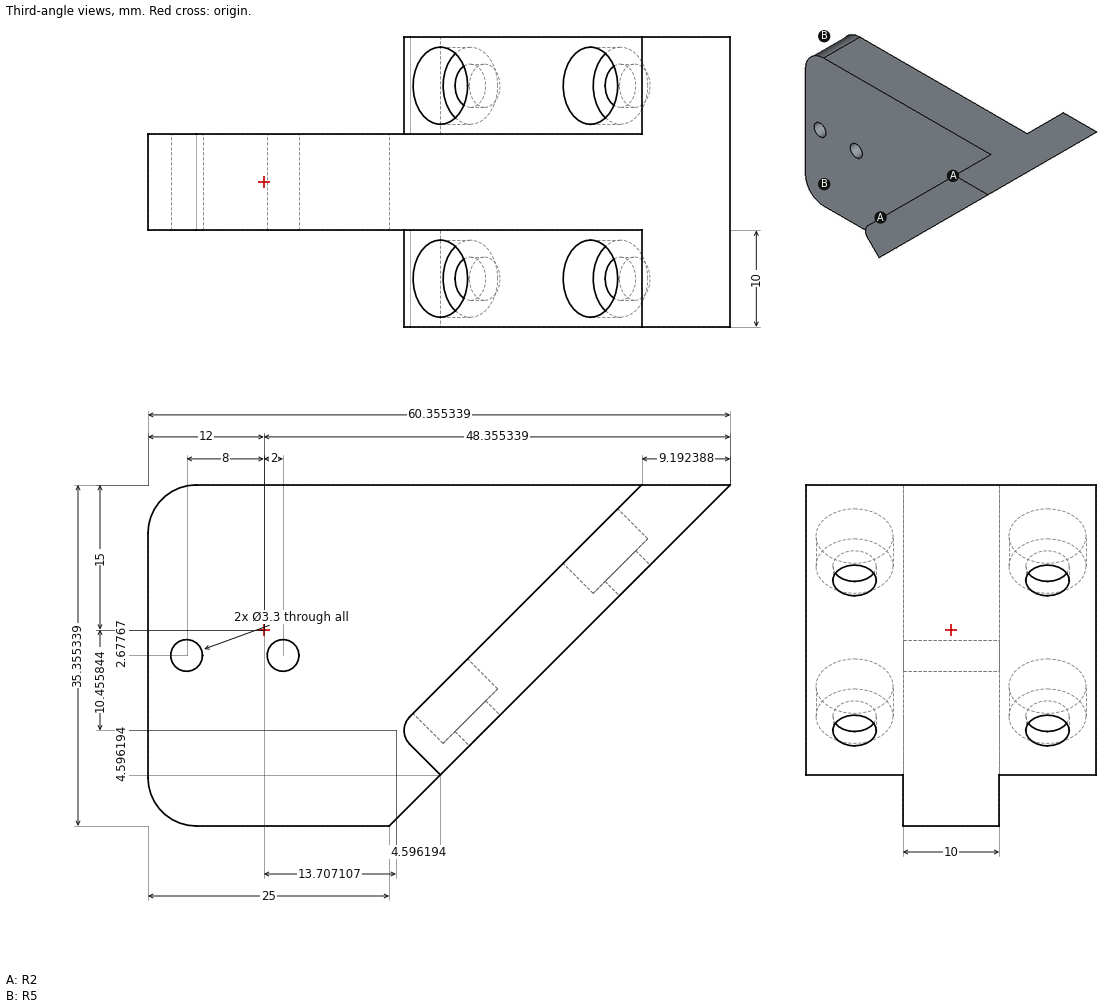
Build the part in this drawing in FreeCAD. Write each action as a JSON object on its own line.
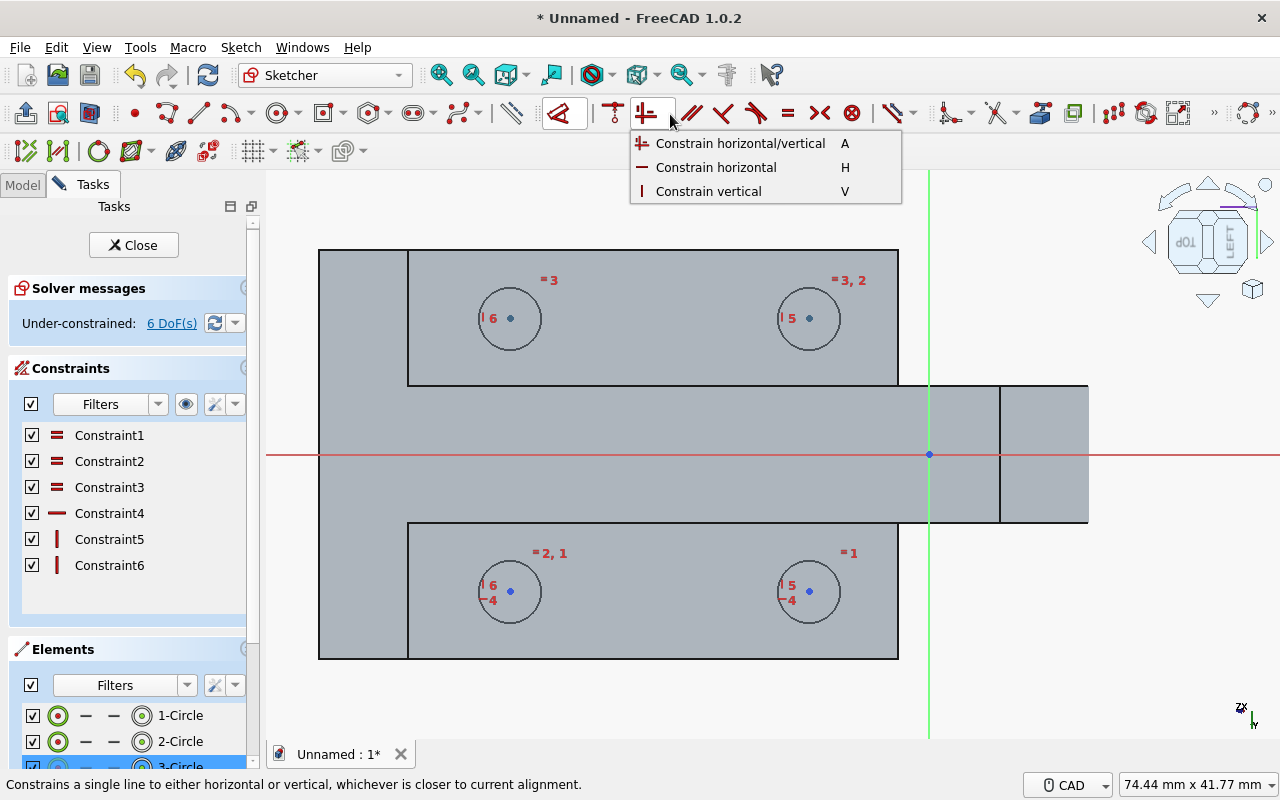
{"action": "left_click", "coordinate": [766, 167]}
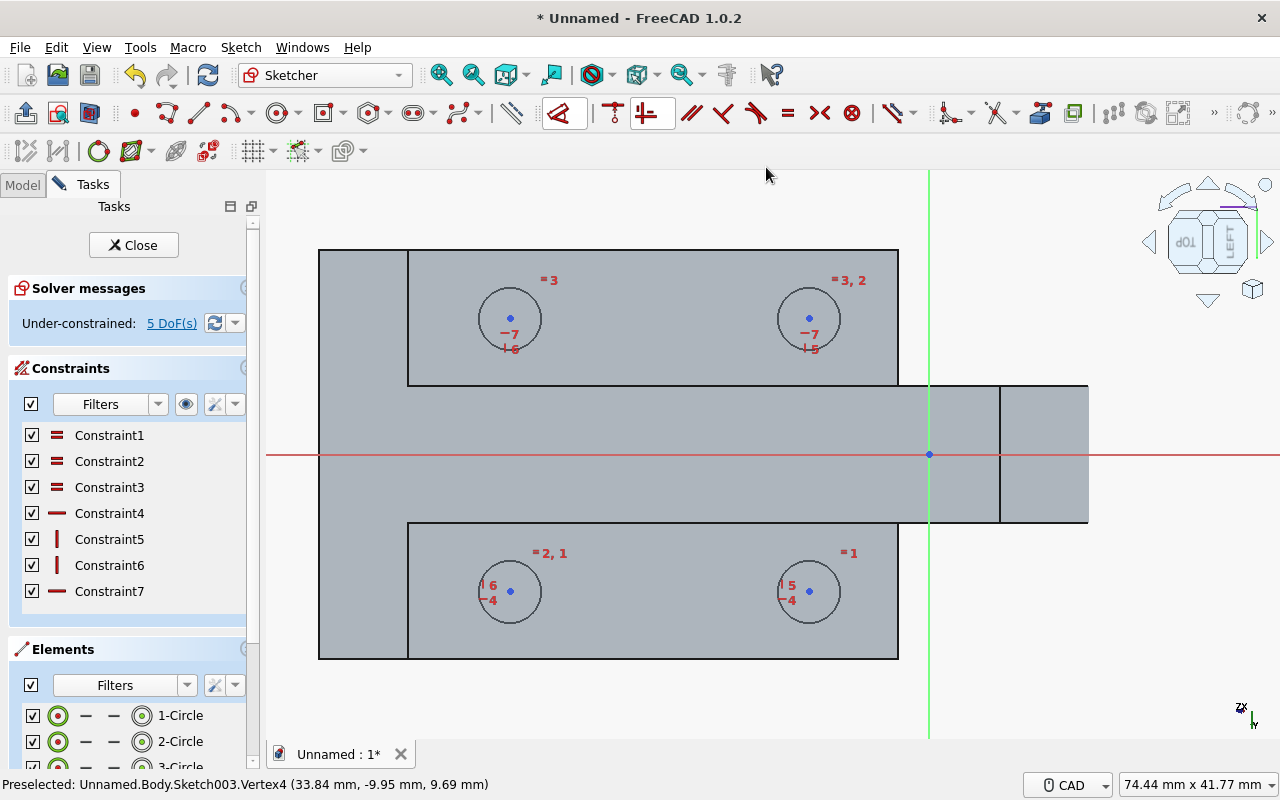
{"action": "left_click", "coordinate": [831, 570]}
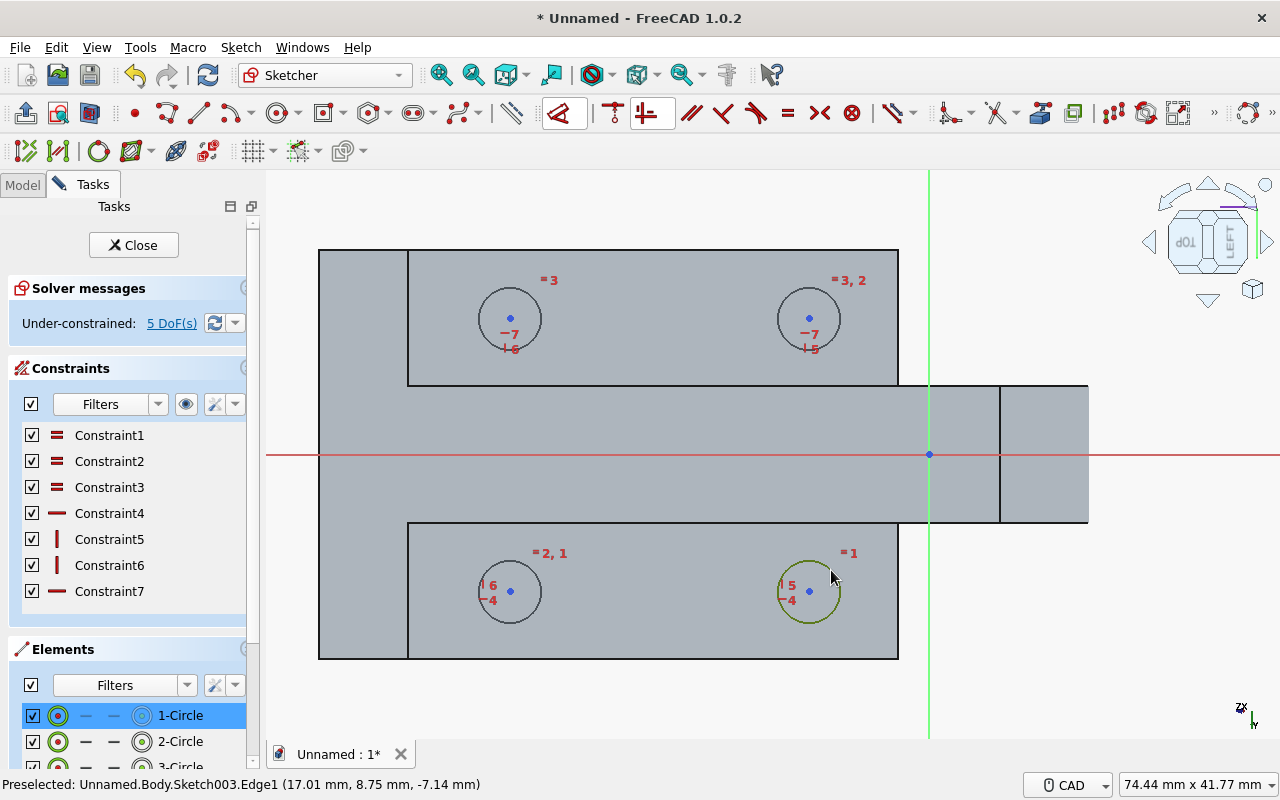
{"action": "key", "text": "k o"}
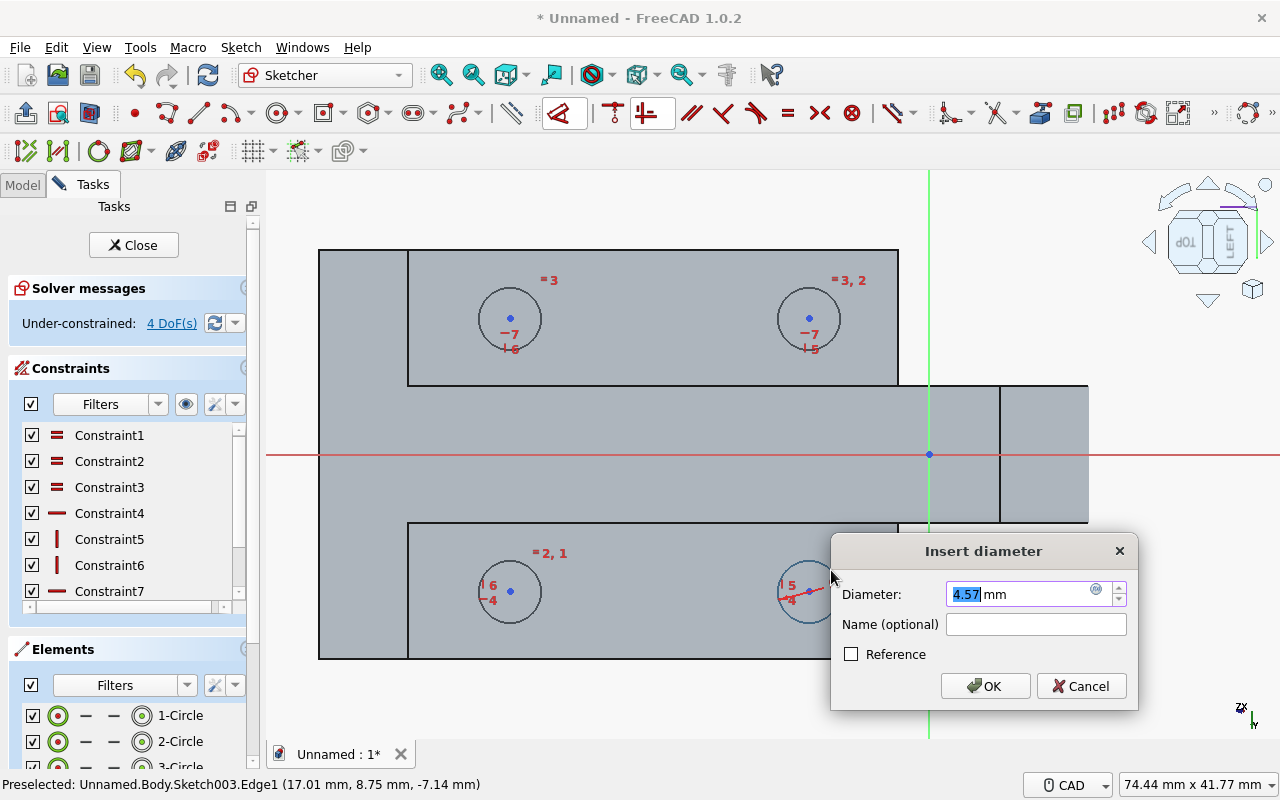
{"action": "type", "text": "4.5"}
{"action": "key", "text": "Return"}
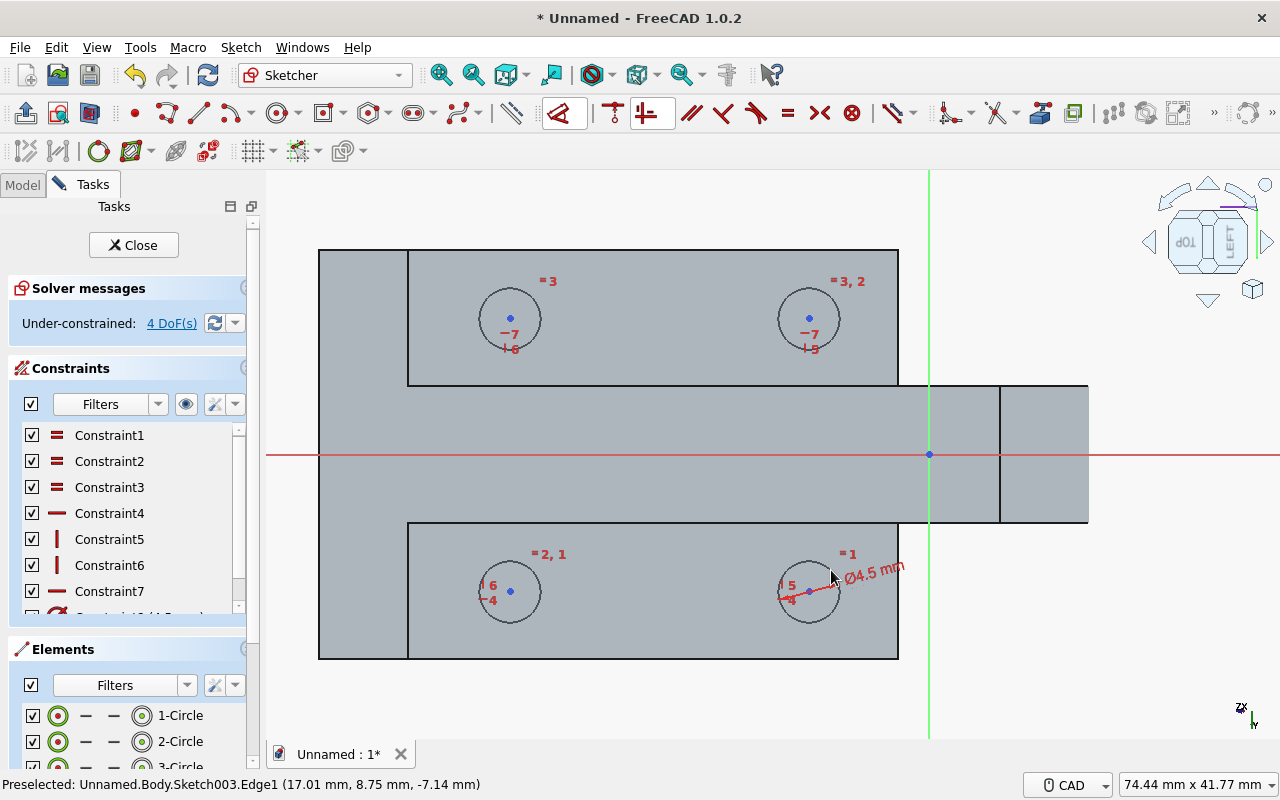
{"action": "left_click", "coordinate": [809, 592]}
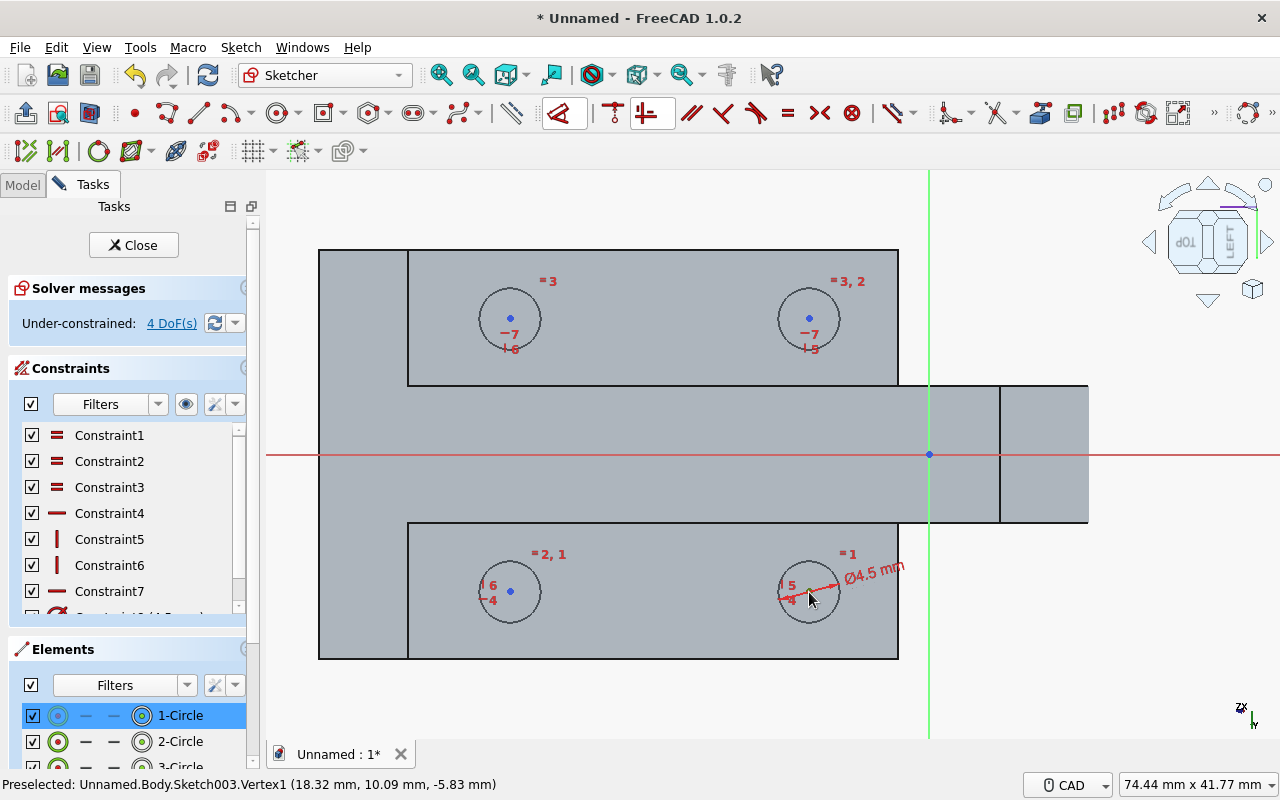
{"action": "left_click", "coordinate": [582, 114]}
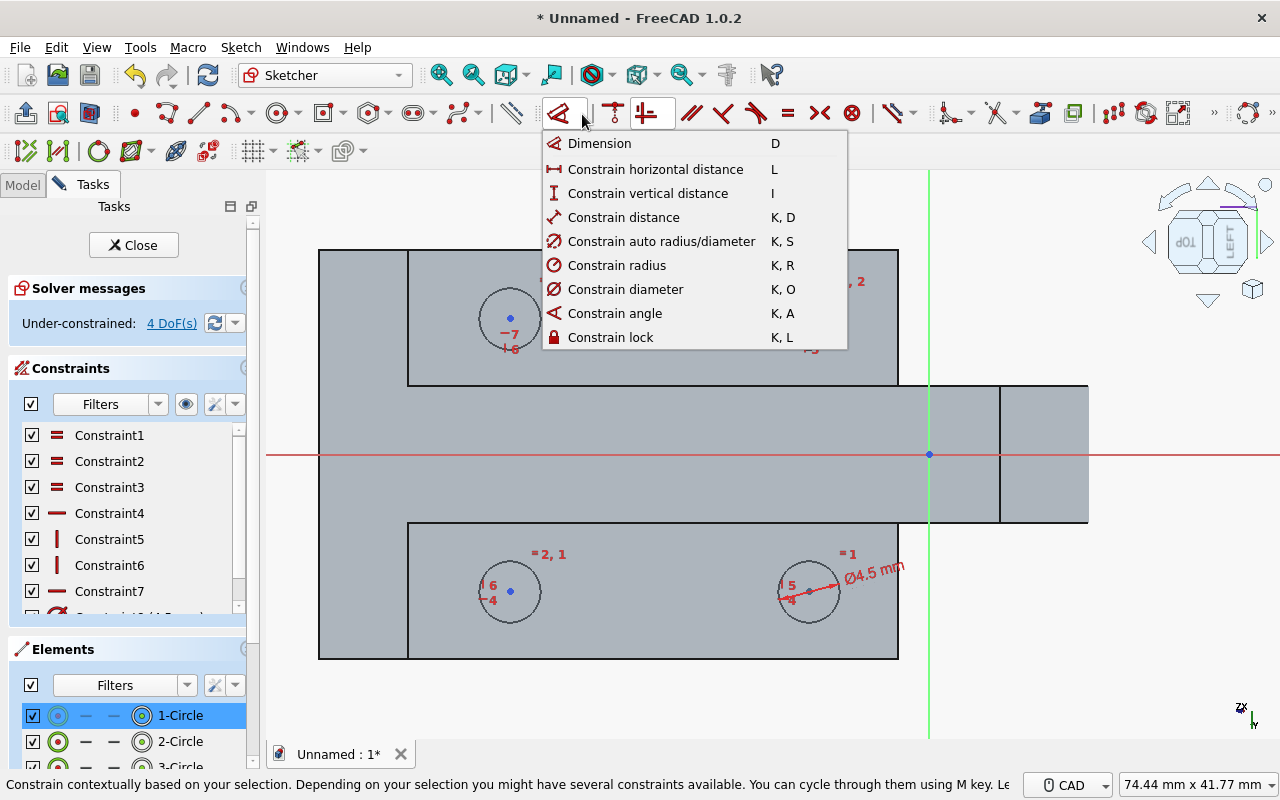
{"action": "left_click", "coordinate": [695, 193]}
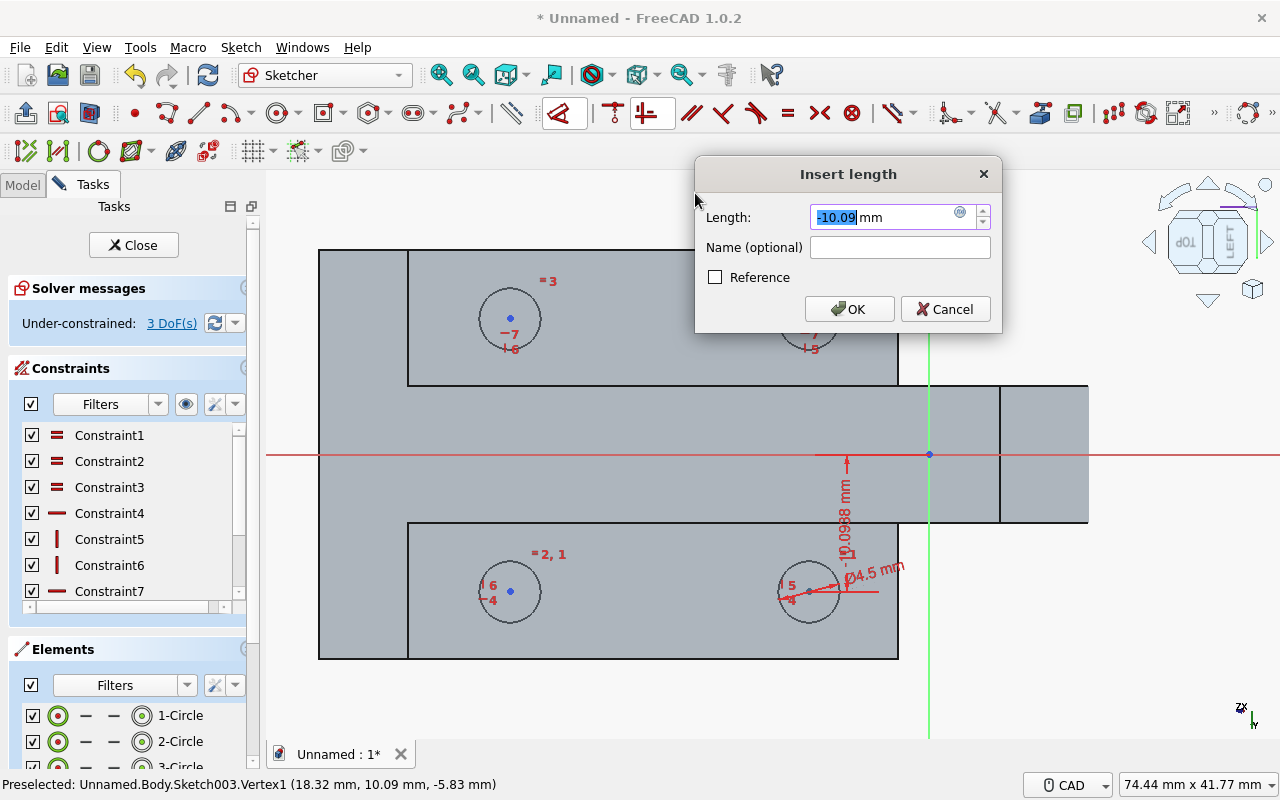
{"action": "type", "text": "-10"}
{"action": "key", "text": "Return"}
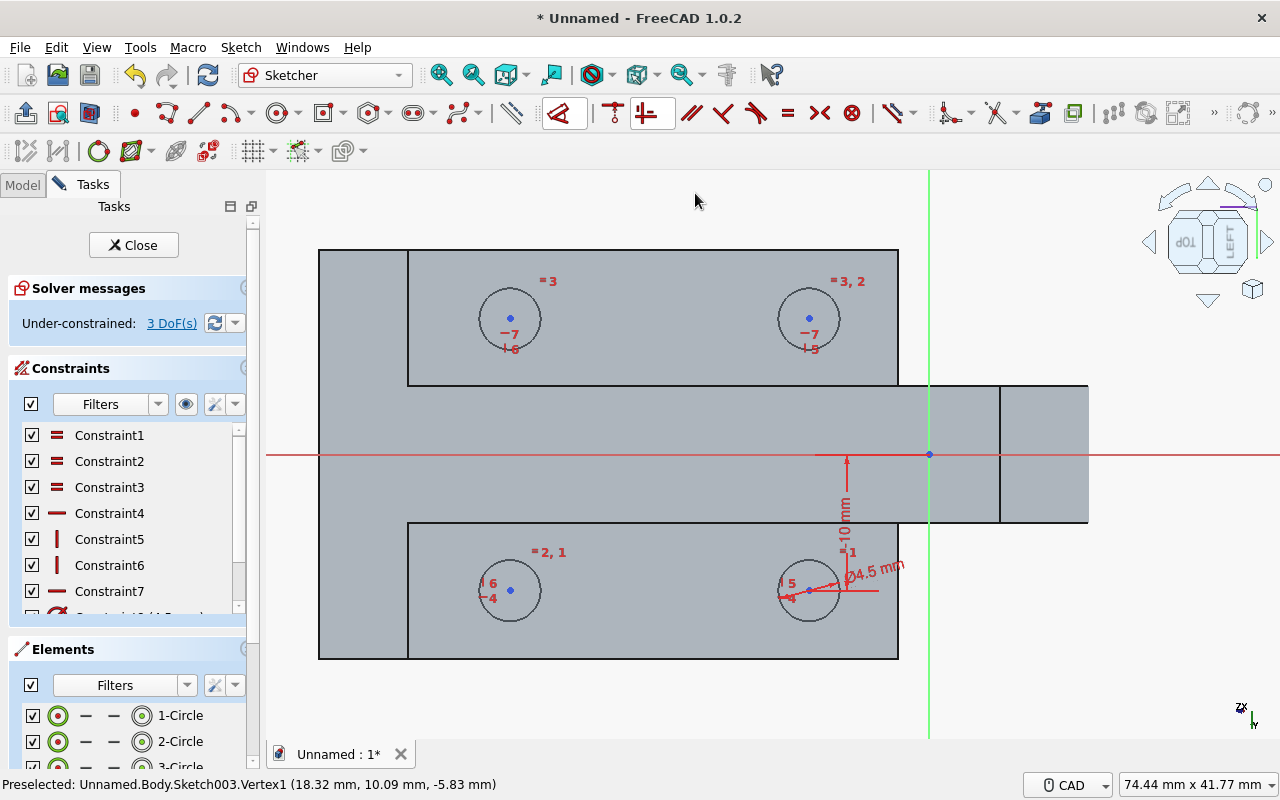
{"action": "left_click", "coordinate": [809, 319]}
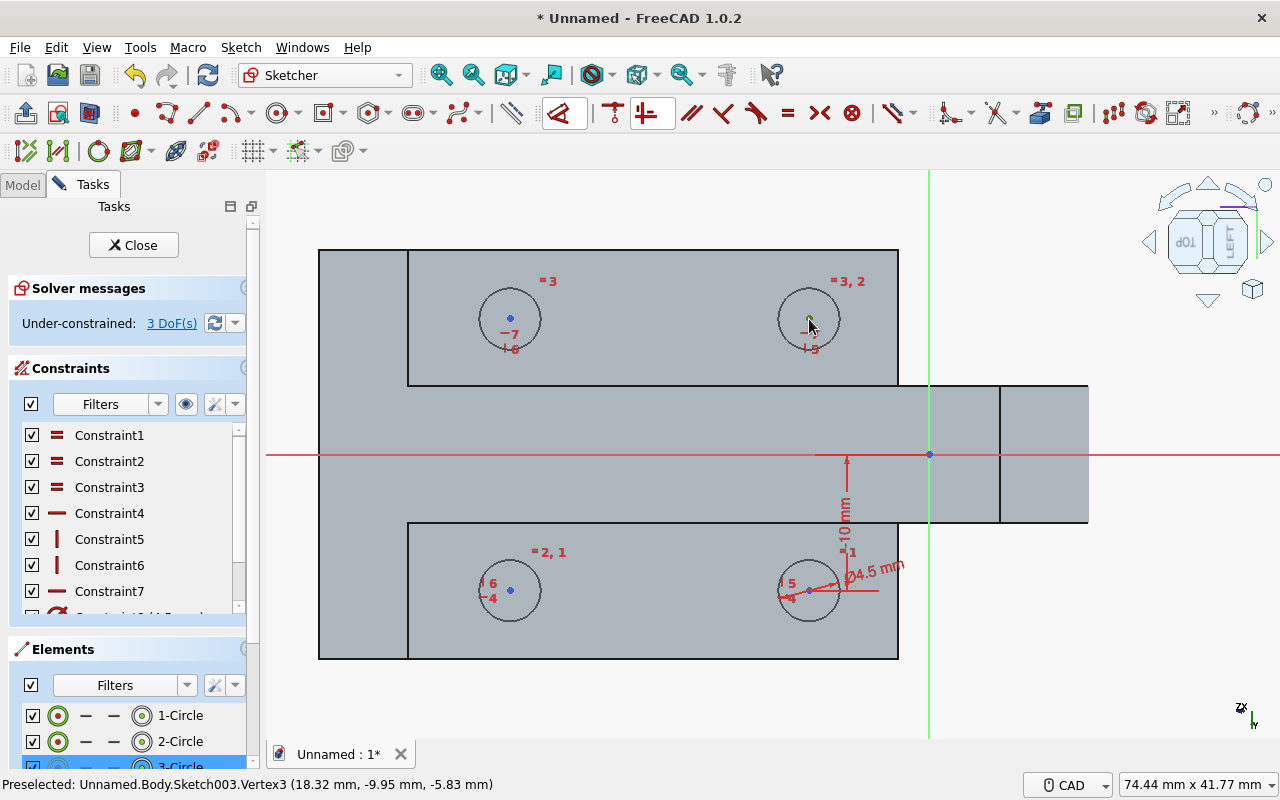
{"action": "key", "text": "i"}